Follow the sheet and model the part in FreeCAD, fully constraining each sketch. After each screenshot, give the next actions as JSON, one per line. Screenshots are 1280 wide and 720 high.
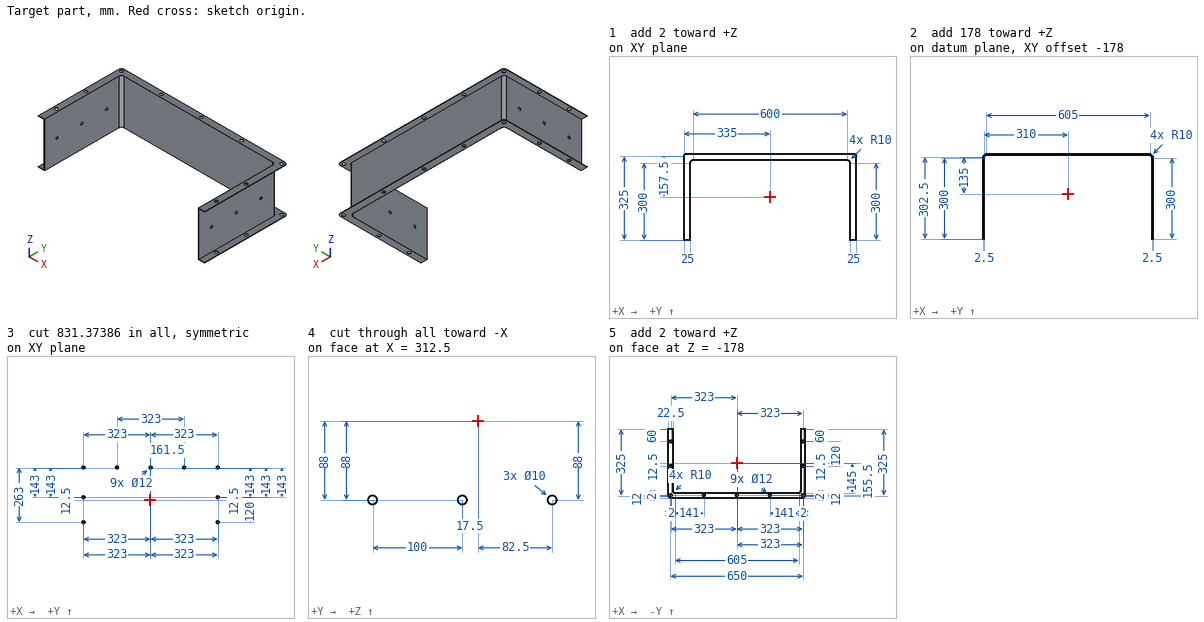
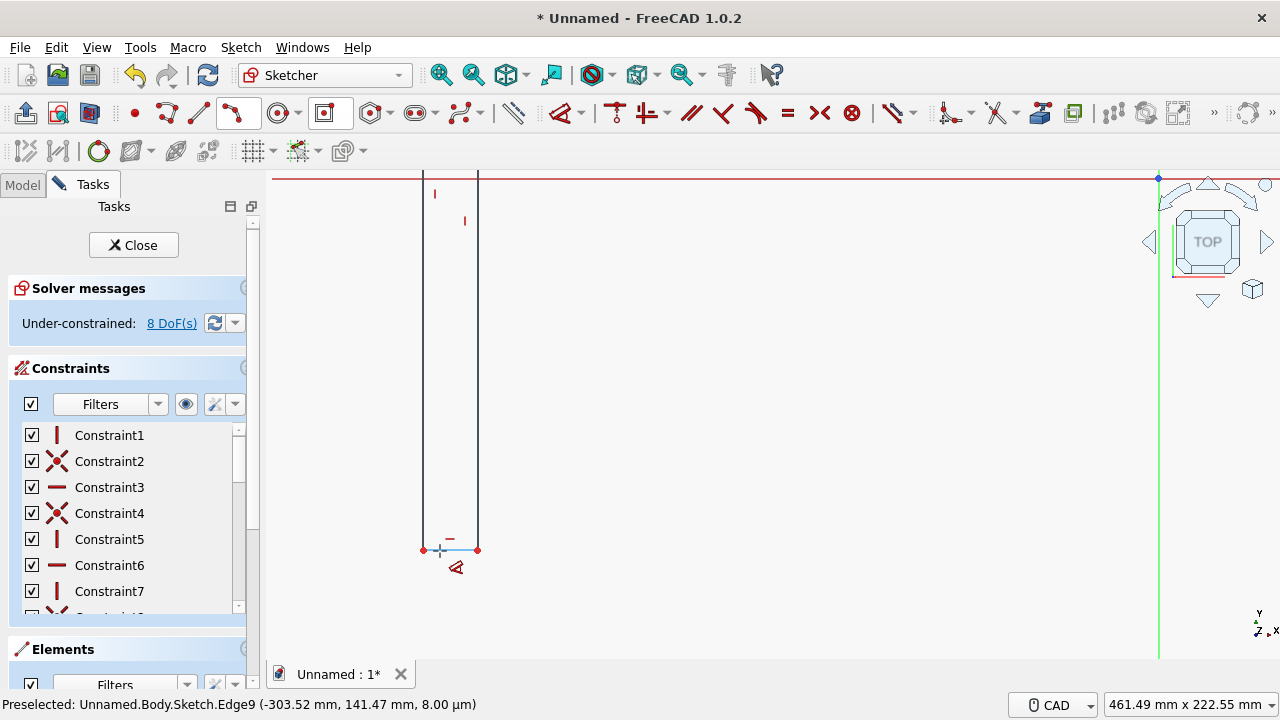
{"action": "left_click", "coordinate": [440, 550]}
{"action": "left_click", "coordinate": [451, 584]}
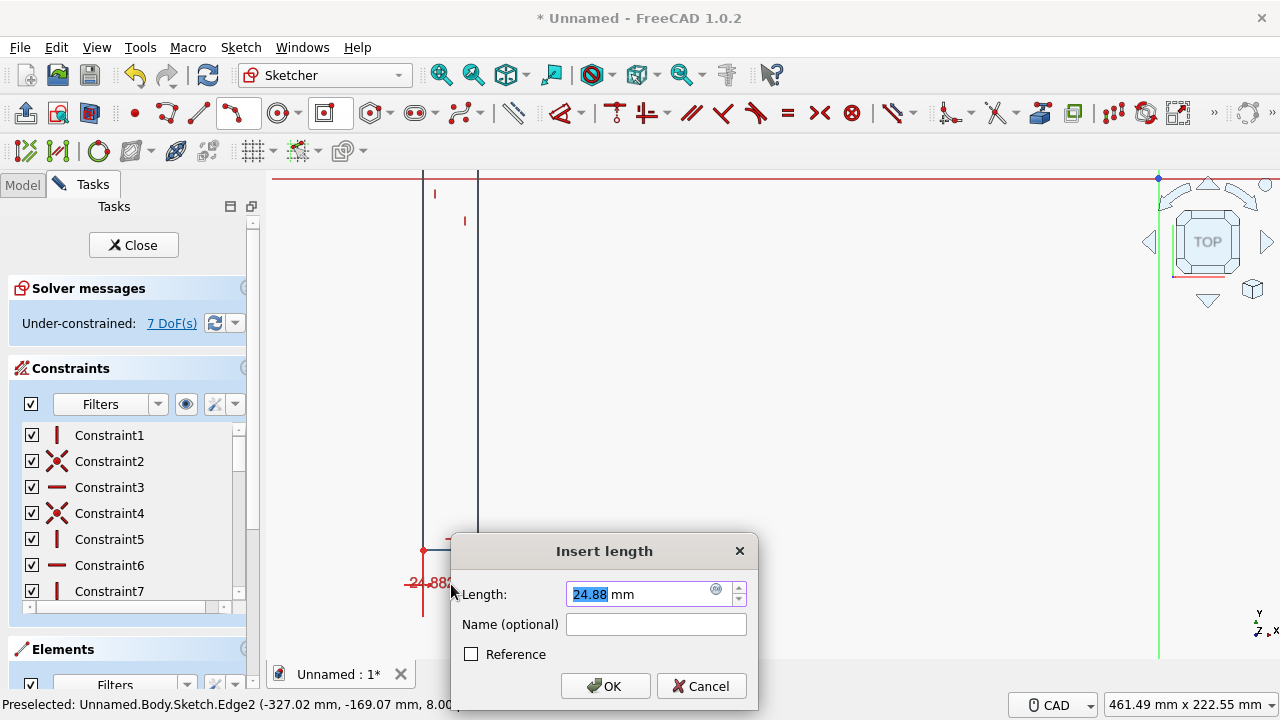
{"action": "type", "text": "25"}
{"action": "key", "text": "Return"}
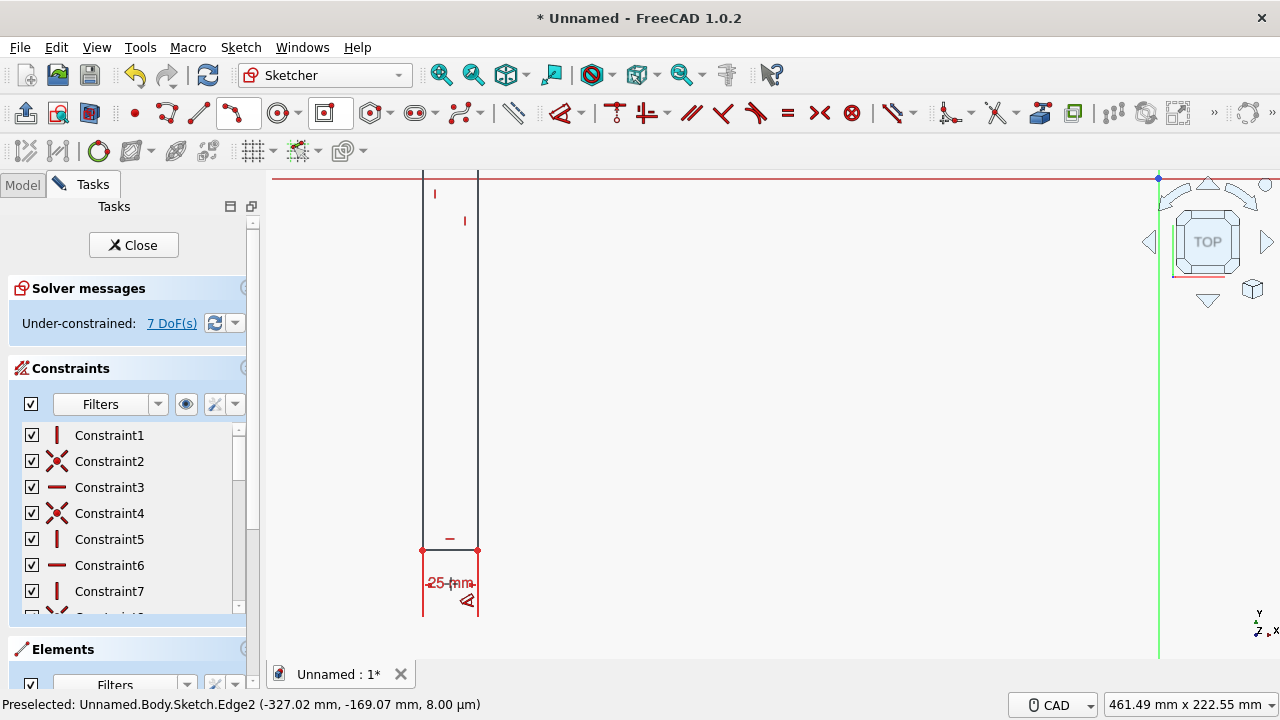
{"action": "scroll", "coordinate": [440, 552], "scroll_direction": "down", "scroll_amount": 5}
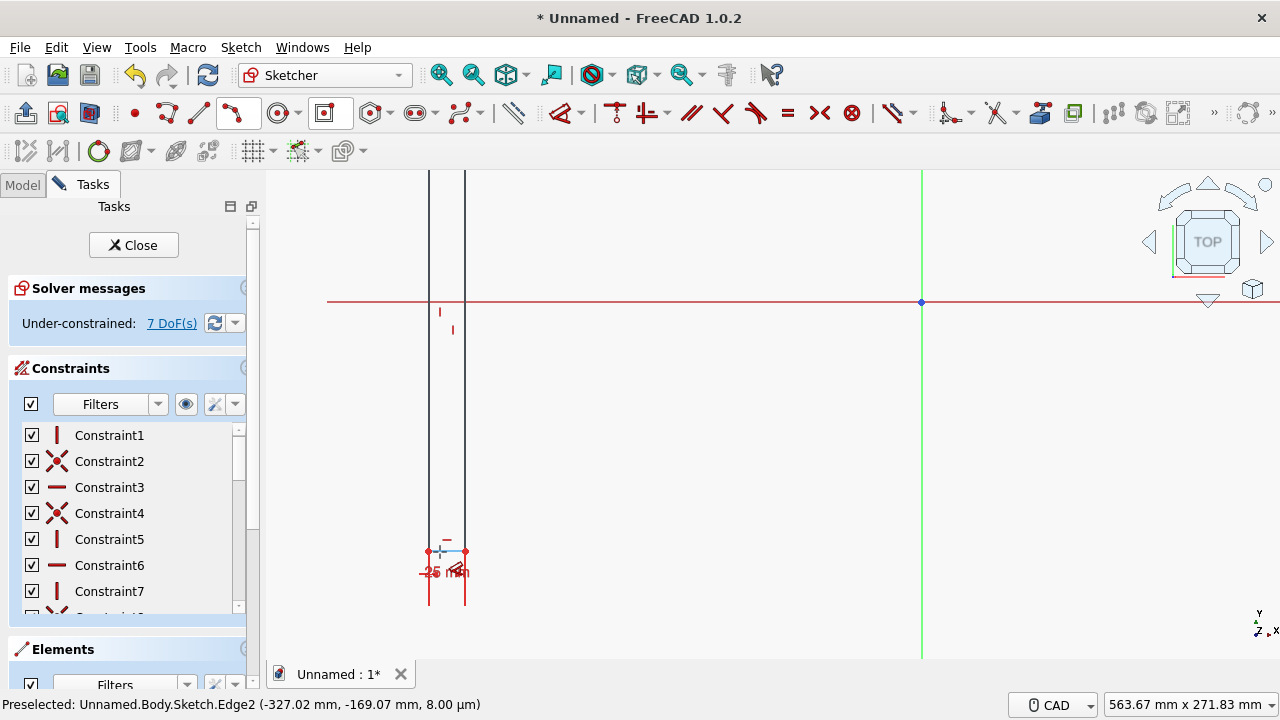
{"action": "scroll", "coordinate": [961, 552], "scroll_direction": "up", "scroll_amount": 5}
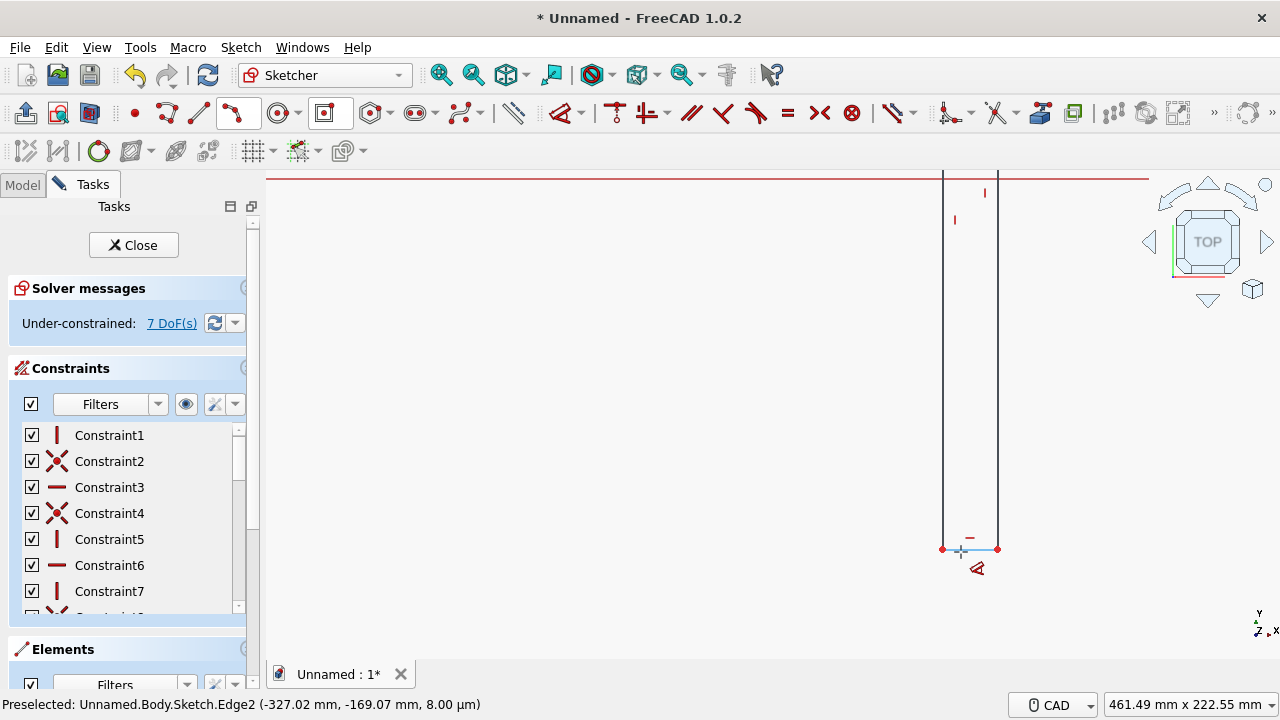
{"action": "left_click", "coordinate": [959, 550]}
{"action": "left_click", "coordinate": [970, 584]}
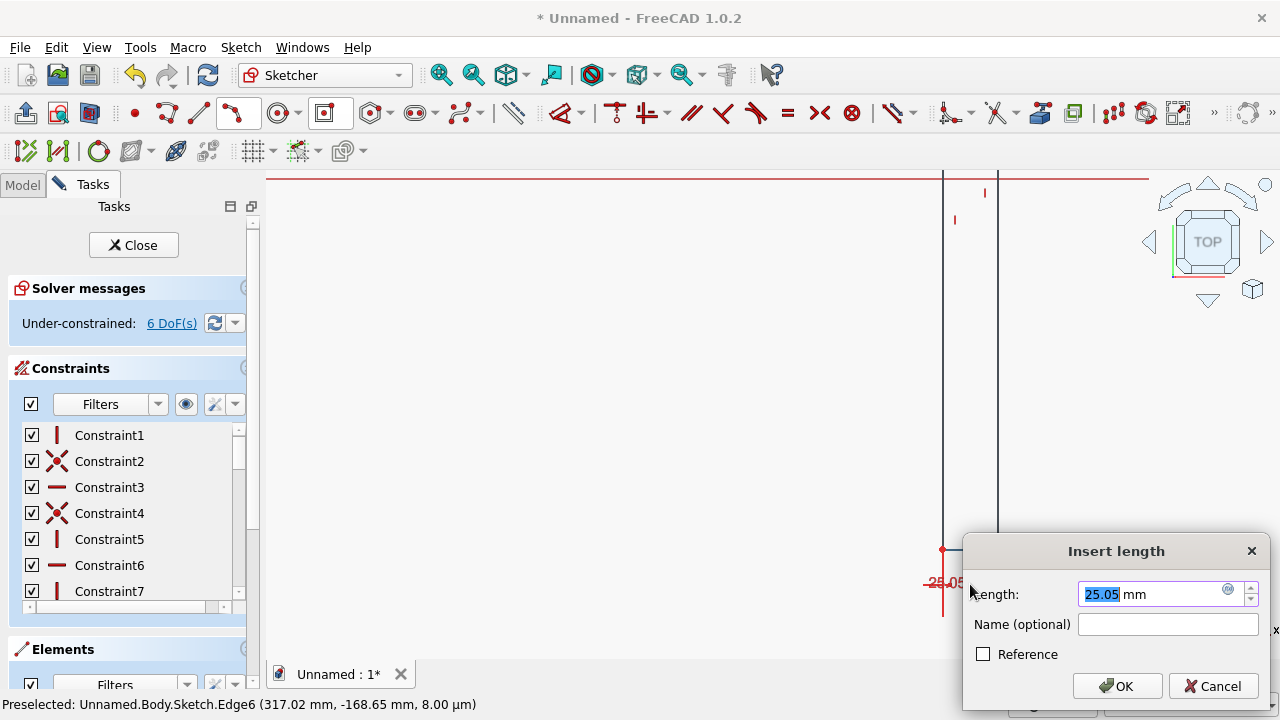
{"action": "type", "text": "25"}
{"action": "key", "text": "Return"}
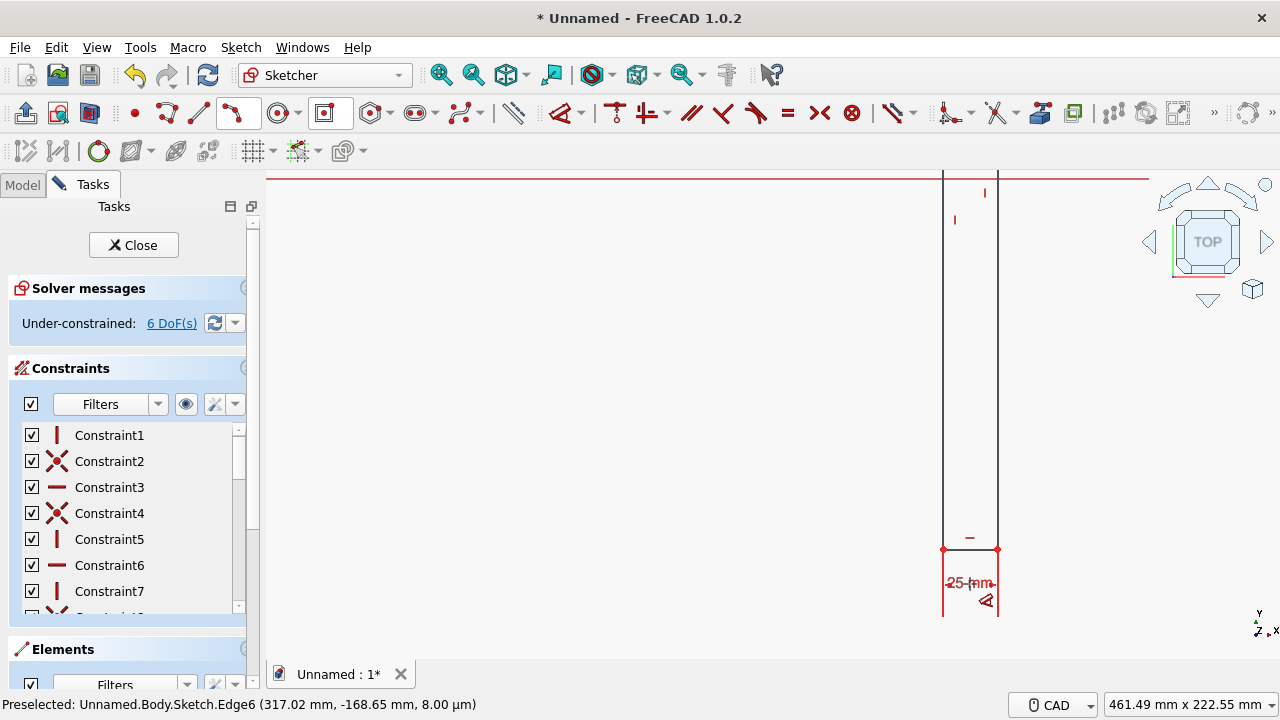
{"action": "scroll", "coordinate": [962, 552], "scroll_direction": "down", "scroll_amount": 5}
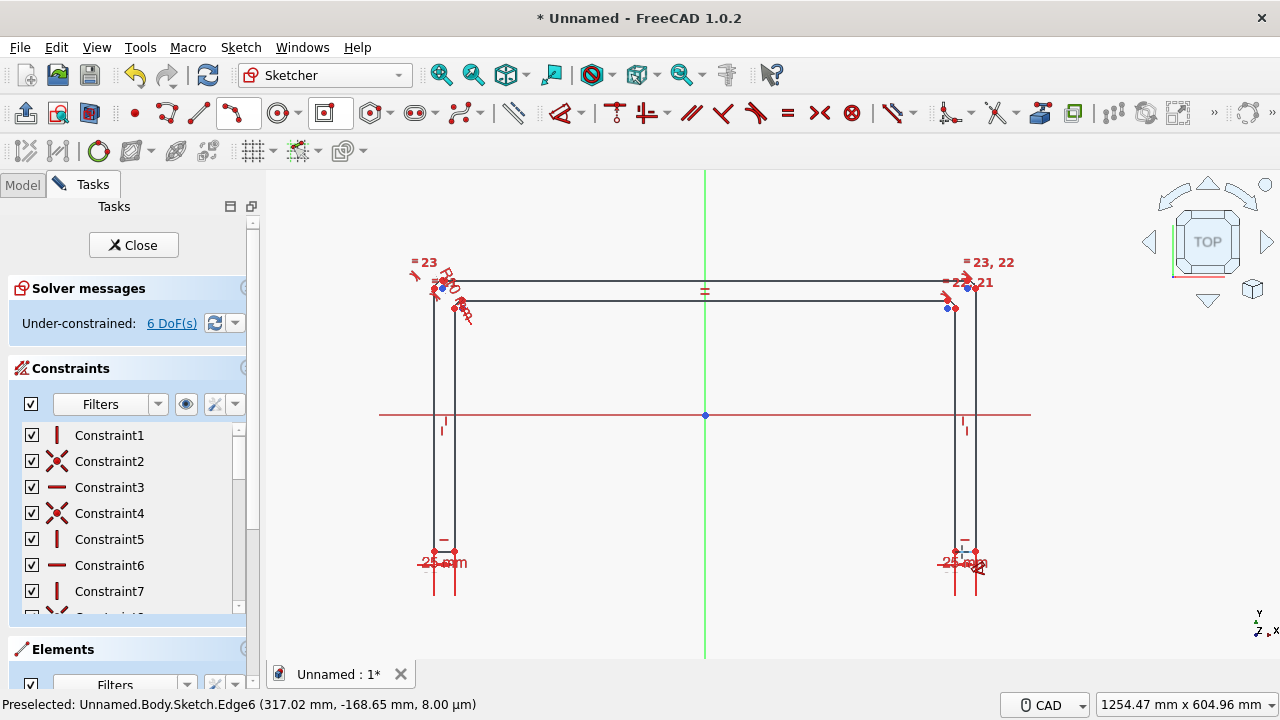
{"action": "left_click", "coordinate": [434, 368]}
{"action": "left_click", "coordinate": [400, 360]}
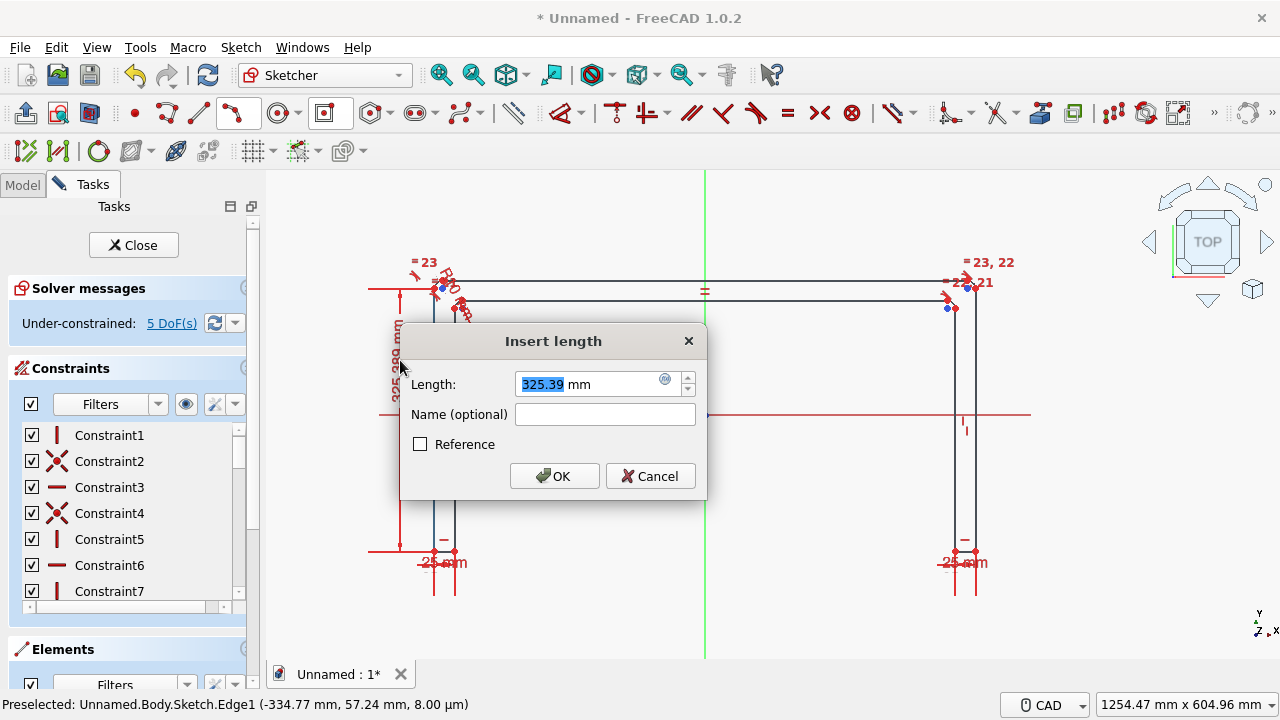
{"action": "type", "text": "325"}
{"action": "key", "text": "Return"}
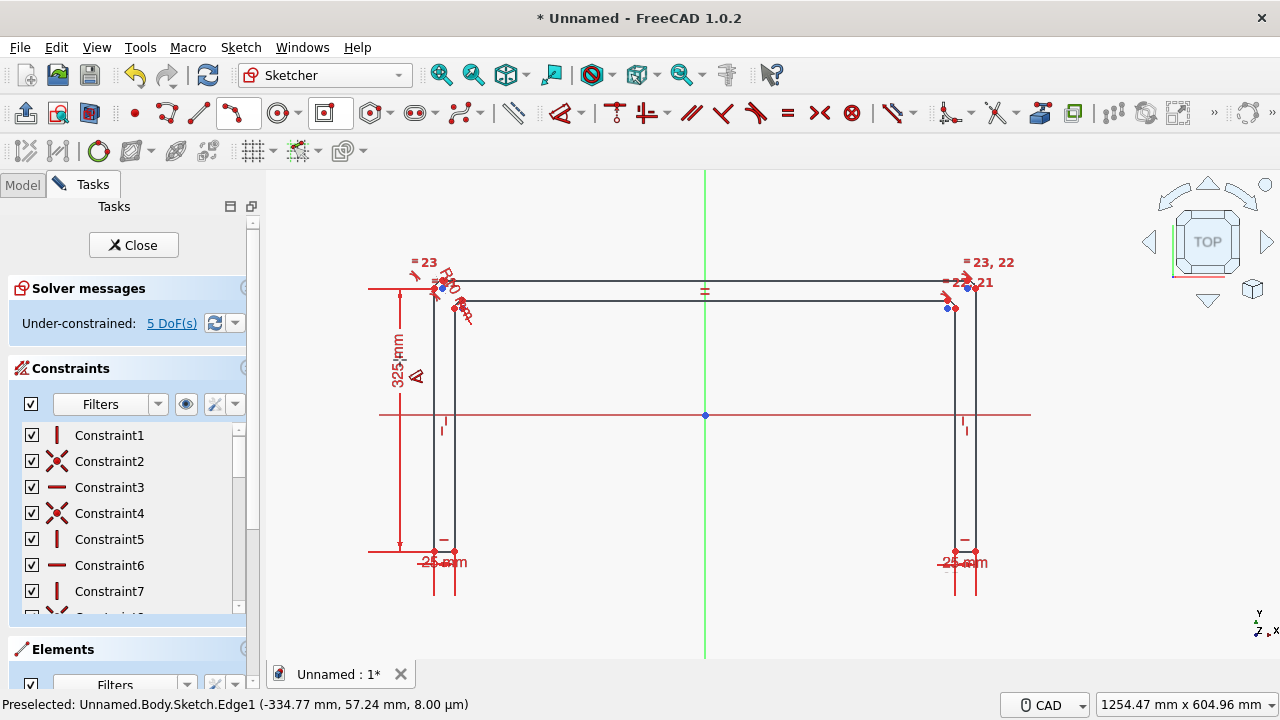
{"action": "left_click", "coordinate": [455, 479]}
{"action": "left_click", "coordinate": [421, 430]}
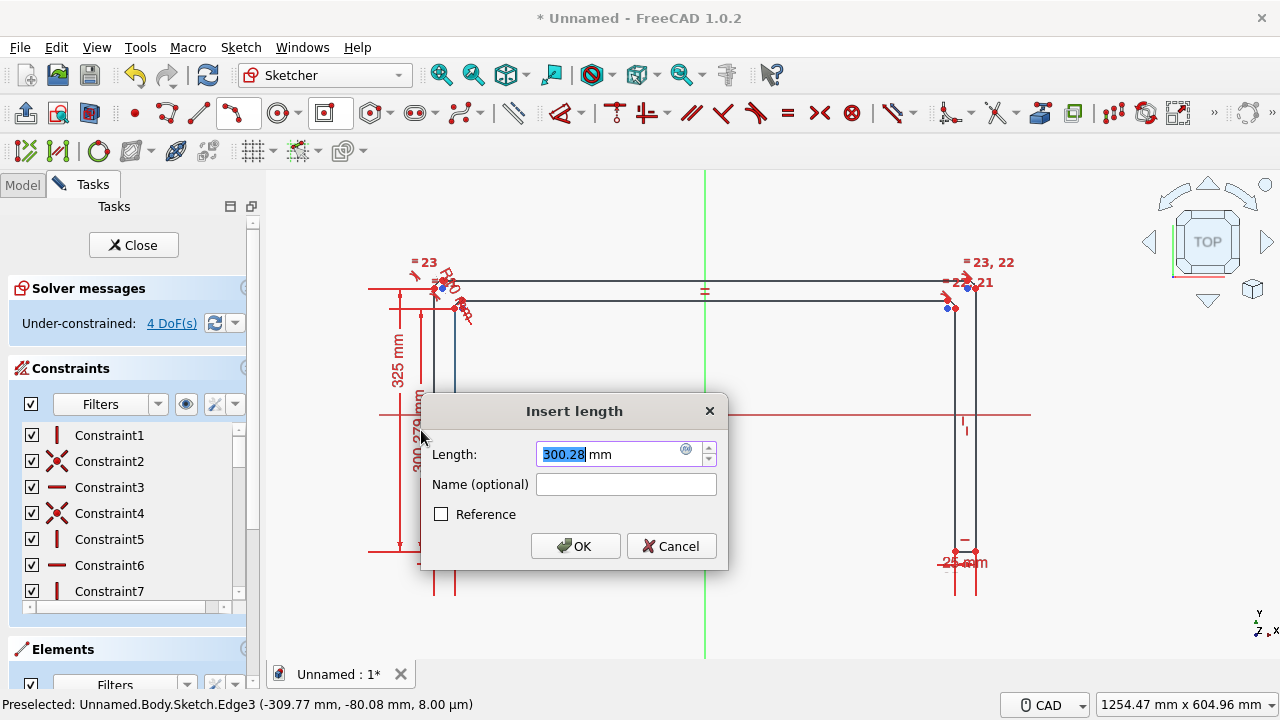
{"action": "type", "text": "300"}
{"action": "key", "text": "Return"}